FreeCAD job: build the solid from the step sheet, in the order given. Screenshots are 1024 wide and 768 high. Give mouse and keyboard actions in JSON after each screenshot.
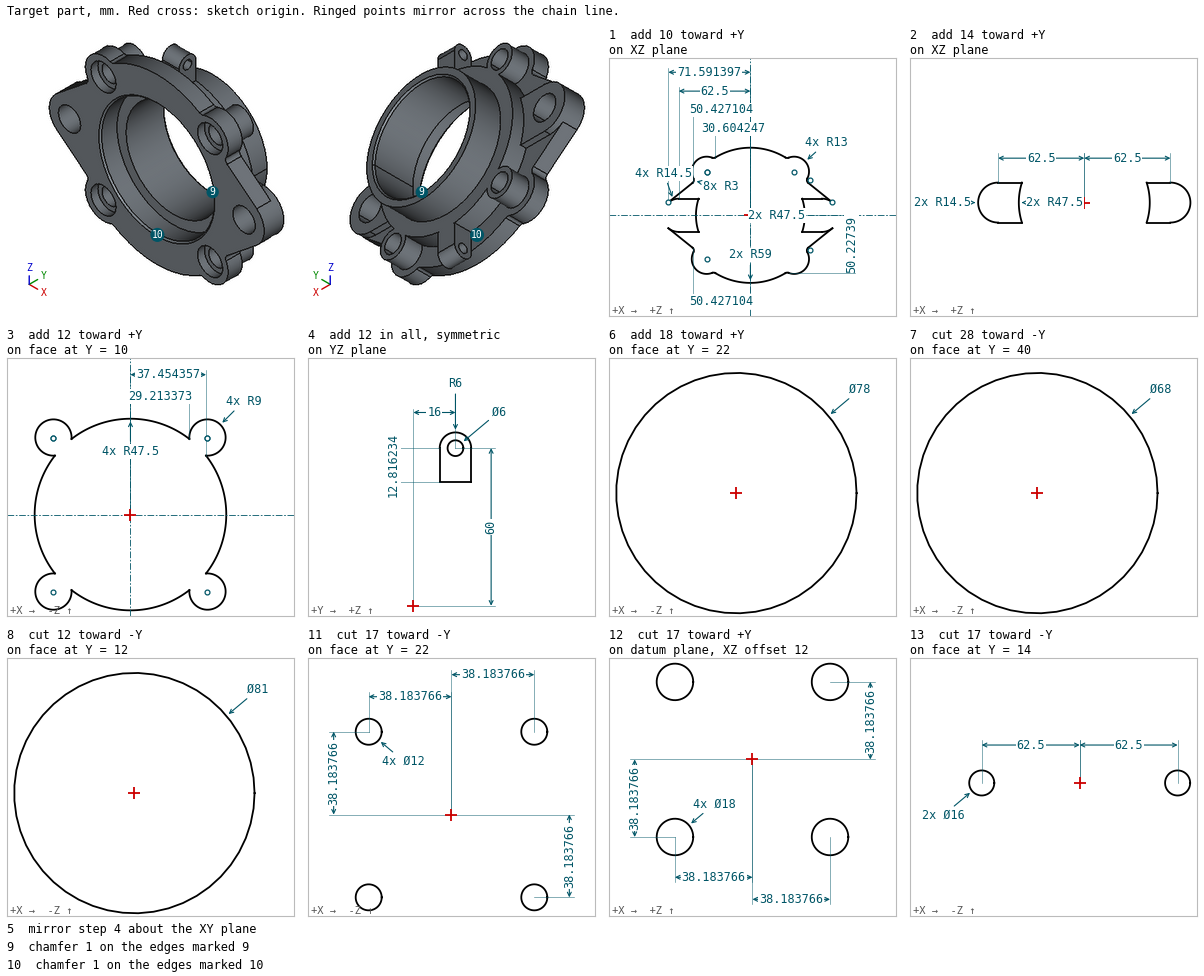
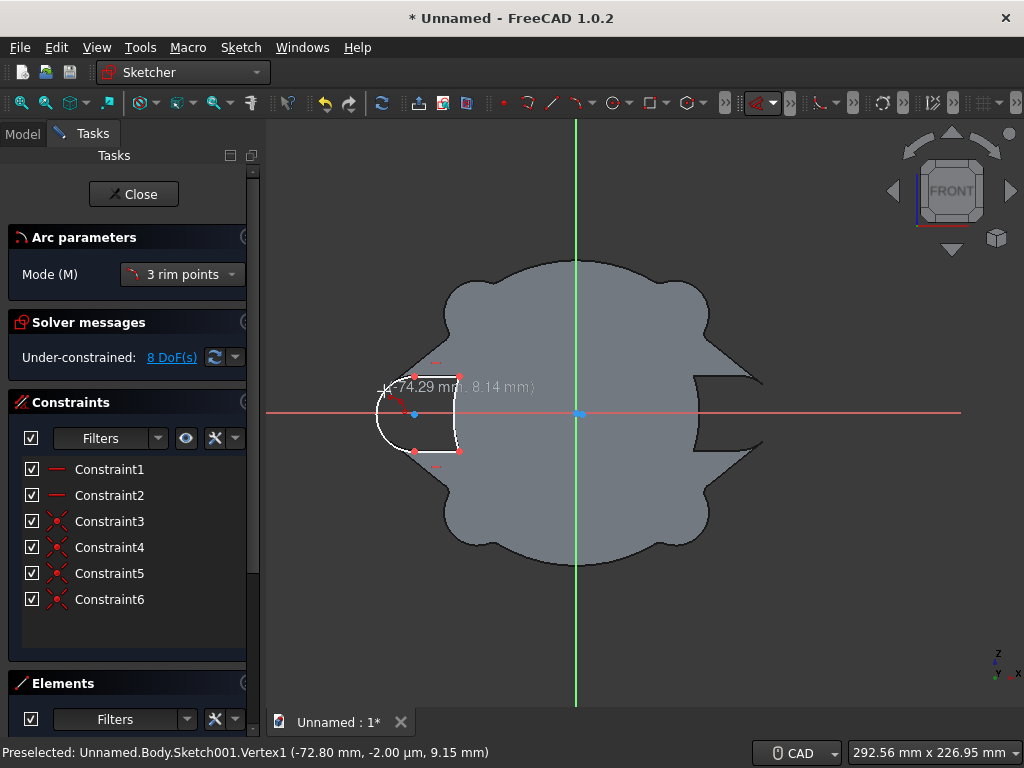
{"action": "key", "text": "g l"}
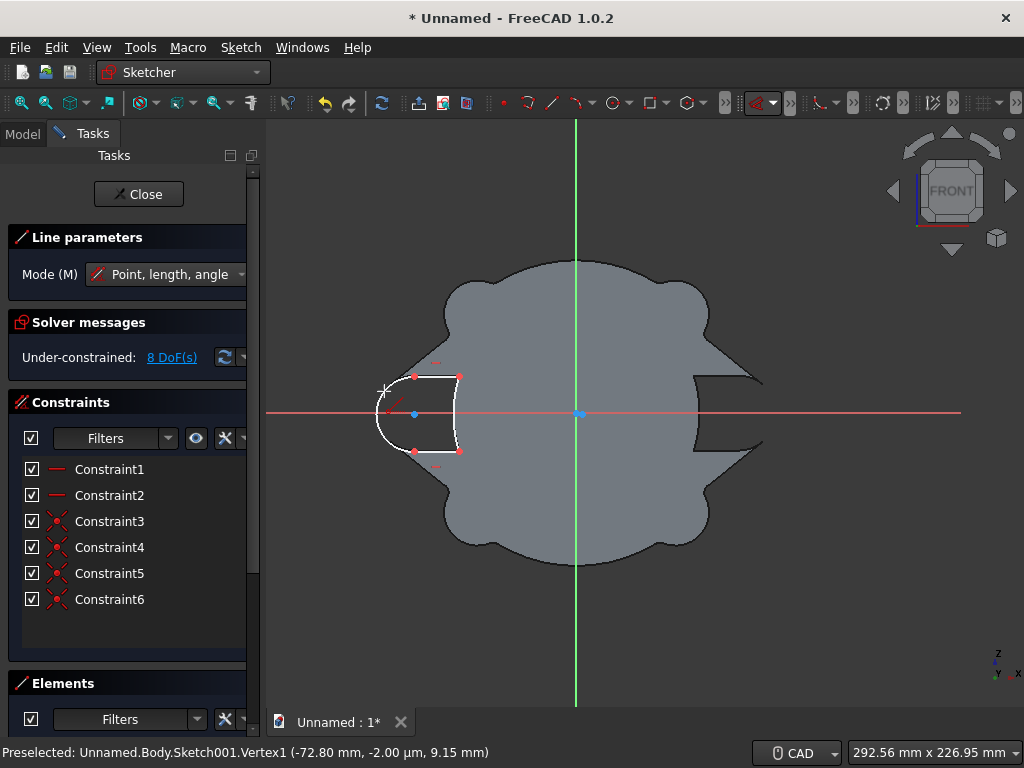
{"action": "left_click", "coordinate": [694, 376]}
{"action": "left_click", "coordinate": [738, 376]}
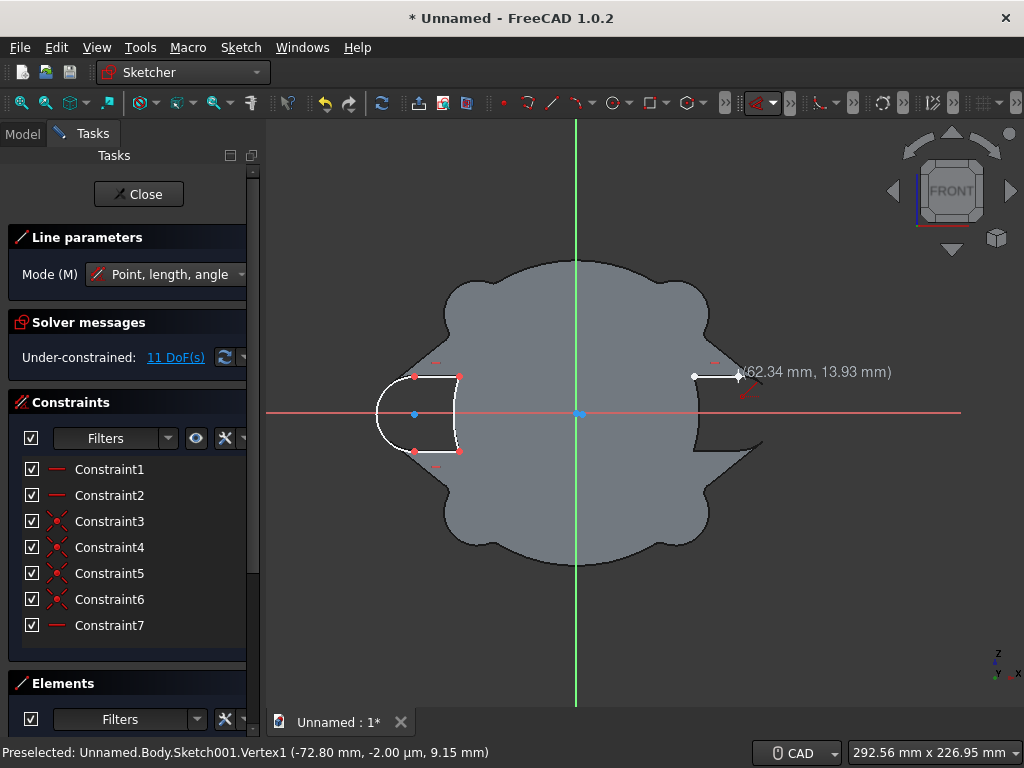
{"action": "left_click", "coordinate": [738, 451]}
{"action": "left_click", "coordinate": [694, 451]}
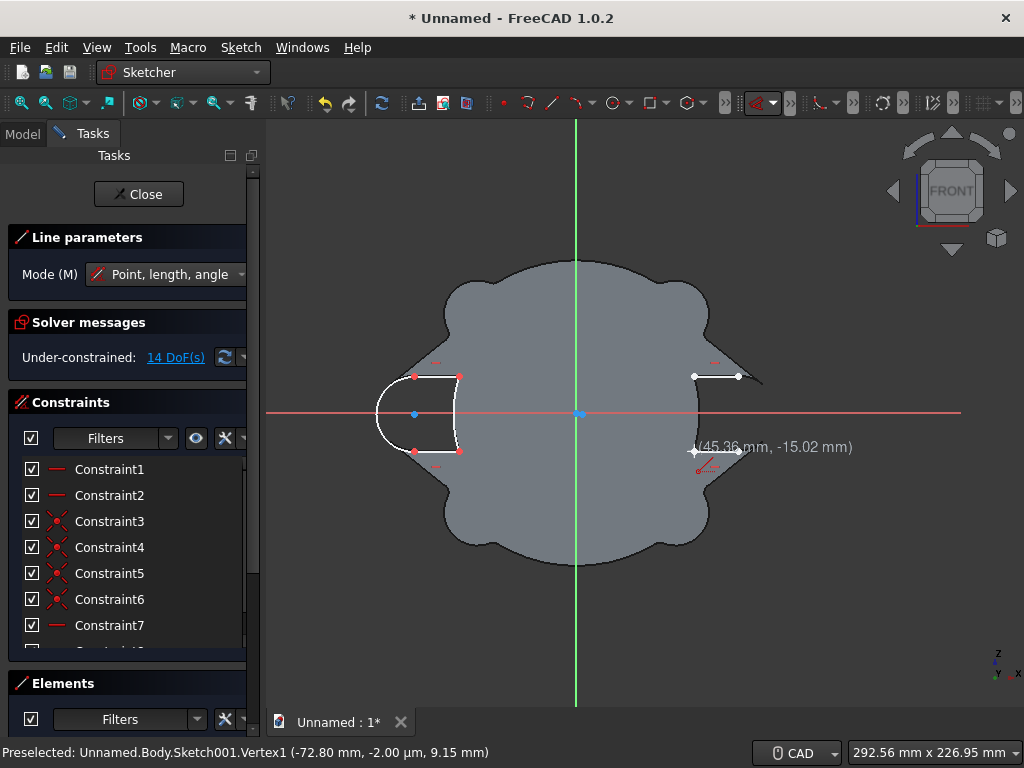
{"action": "key", "text": "g 3 a"}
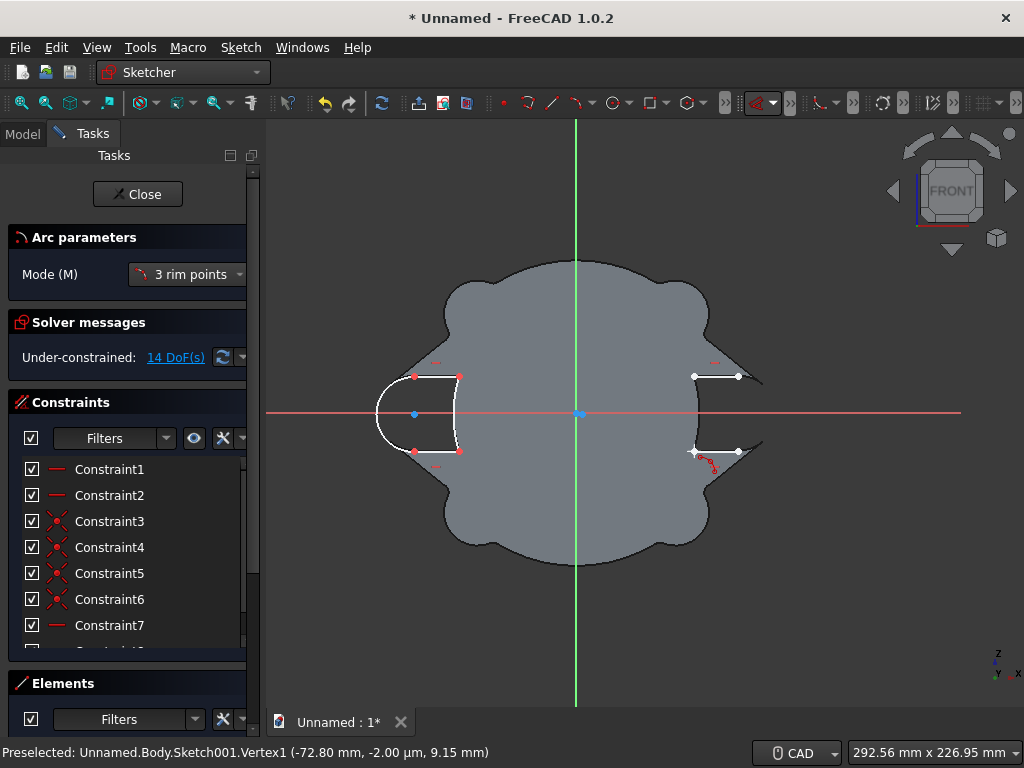
{"action": "left_click", "coordinate": [738, 377]}
{"action": "left_click", "coordinate": [738, 452]}
{"action": "left_click", "coordinate": [769, 435]}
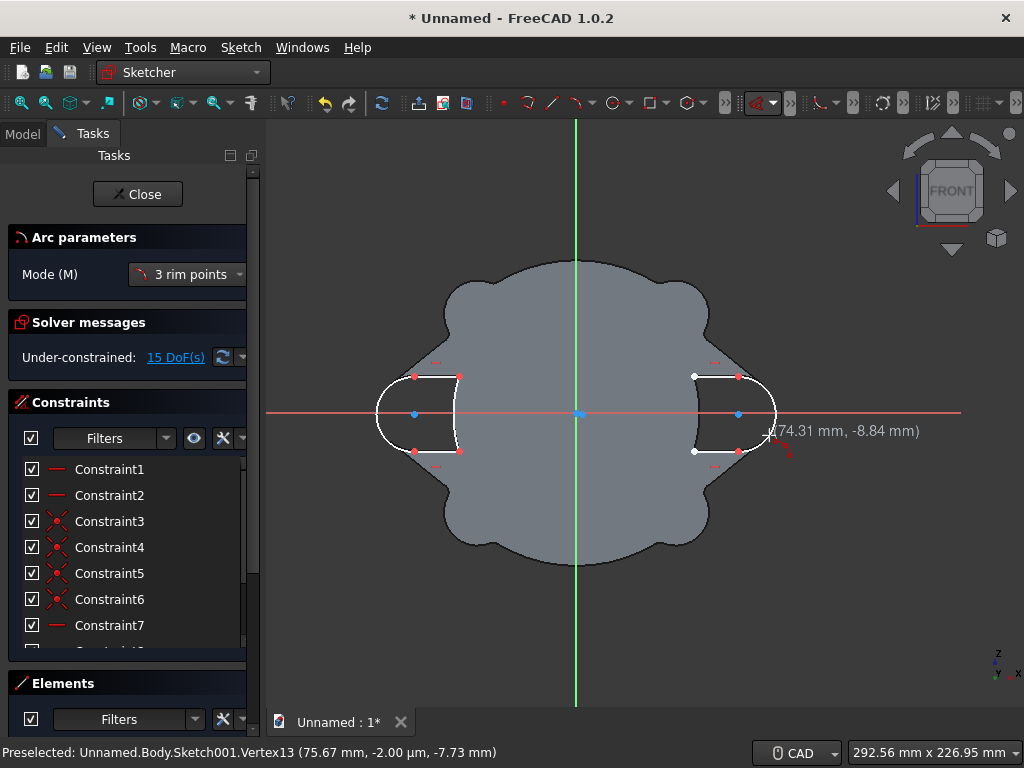
{"action": "left_click", "coordinate": [694, 452]}
{"action": "left_click", "coordinate": [694, 377]}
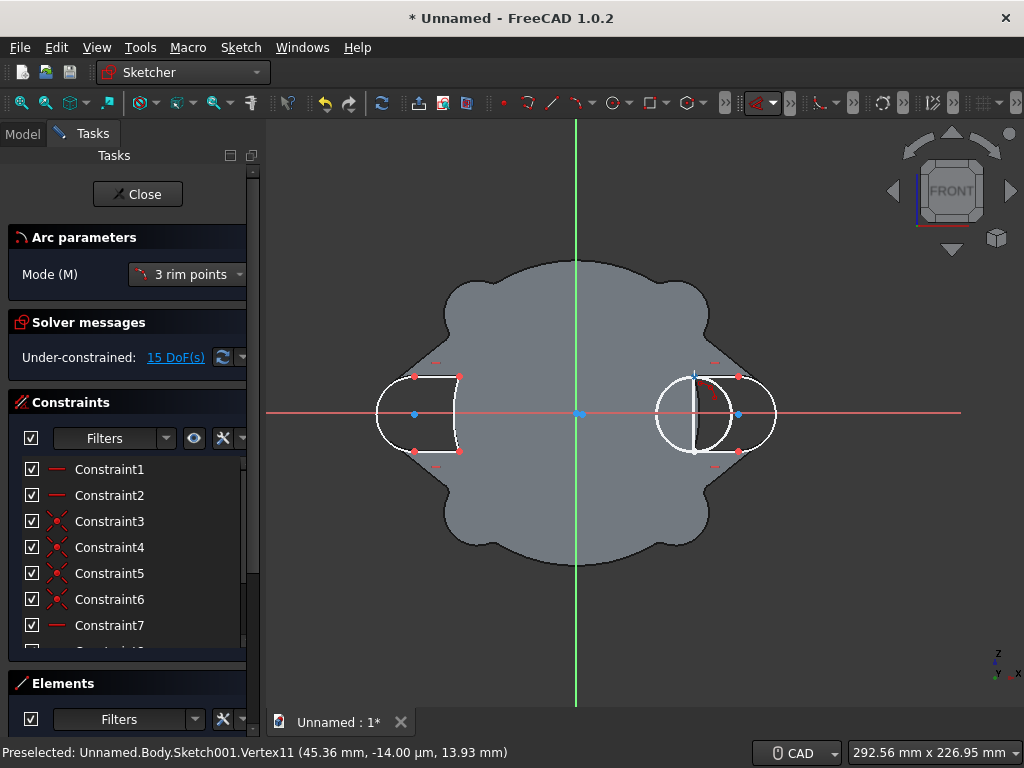
{"action": "scroll", "coordinate": [699, 421], "scroll_direction": "up", "scroll_amount": 6}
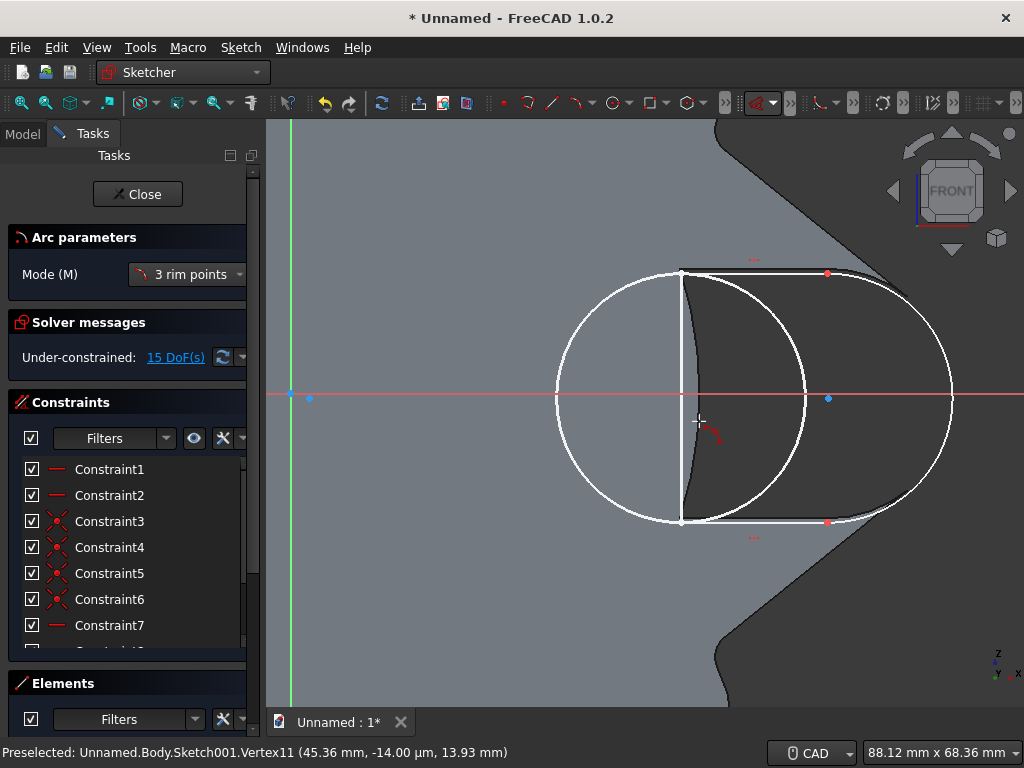
{"action": "left_click", "coordinate": [699, 419]}
{"action": "key", "text": "Escape"}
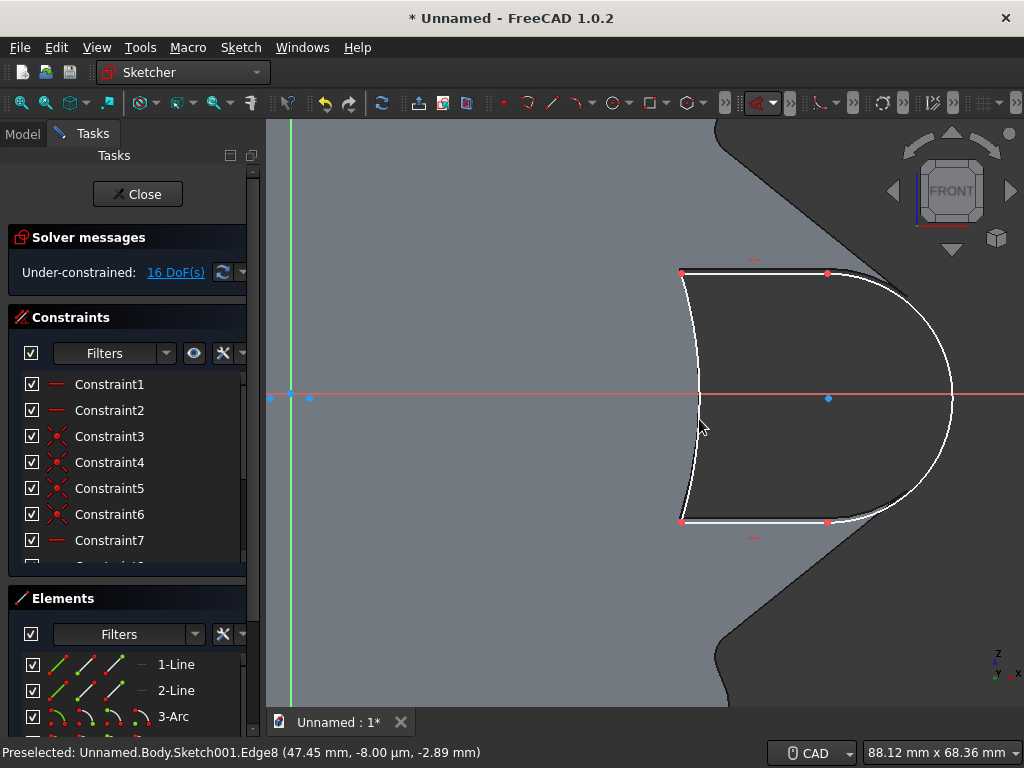
{"action": "scroll", "coordinate": [700, 421], "scroll_direction": "down", "scroll_amount": 6}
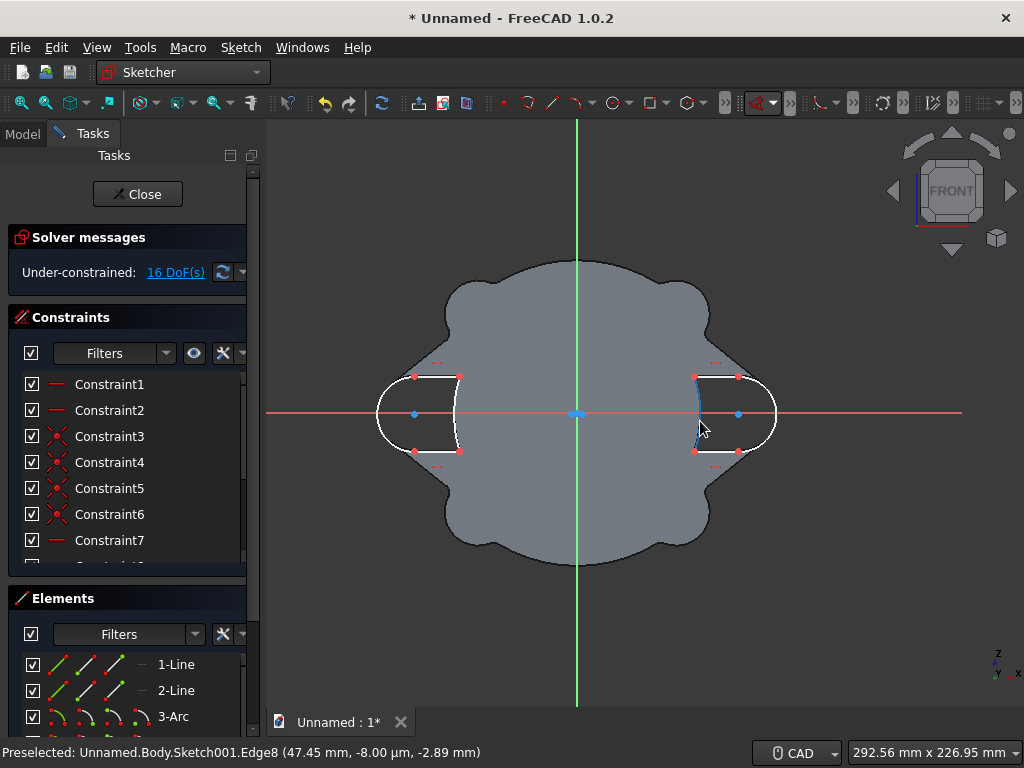
{"action": "left_click", "coordinate": [428, 377]}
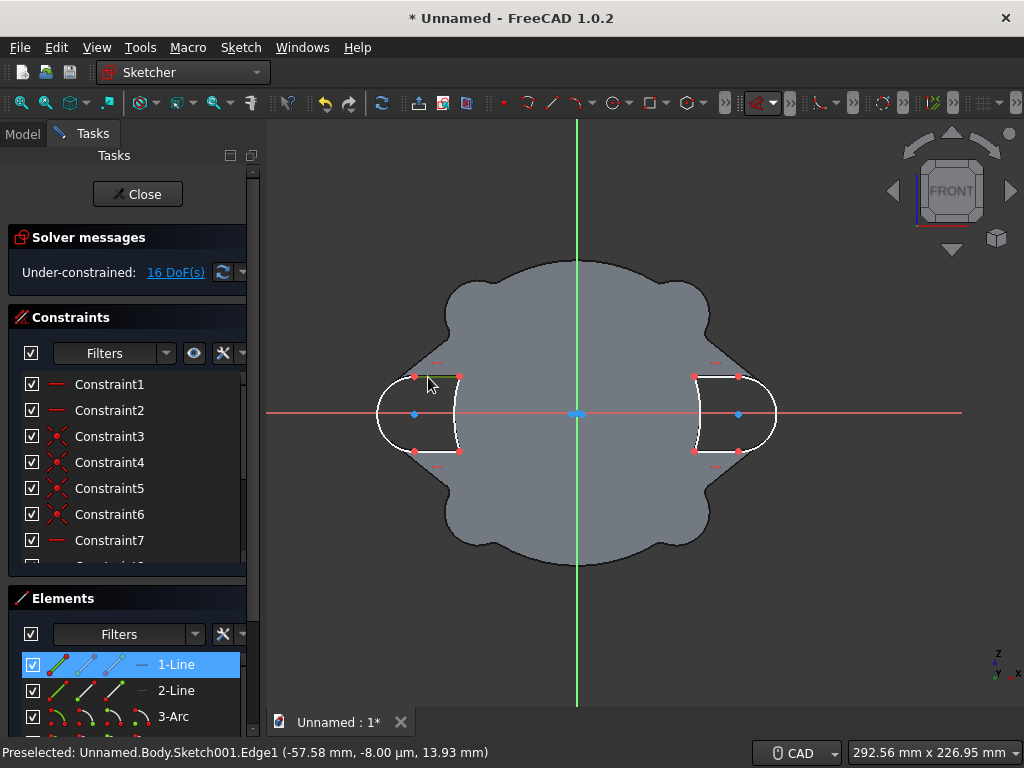
{"action": "left_click", "coordinate": [384, 392]}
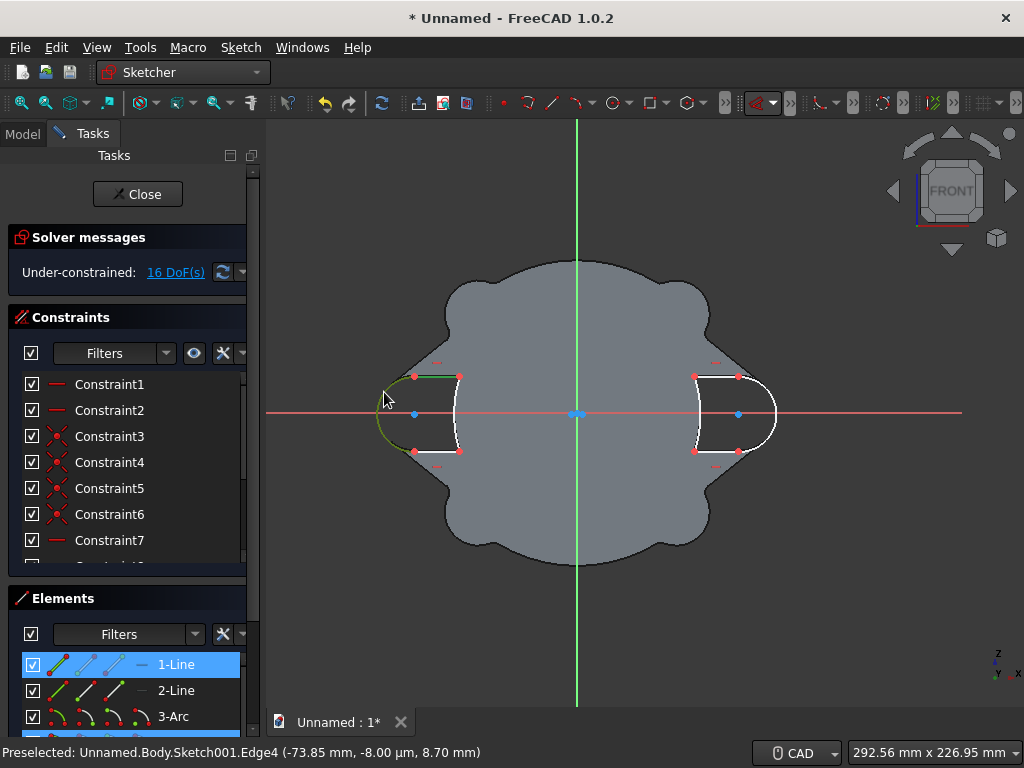
{"action": "key", "text": "t"}